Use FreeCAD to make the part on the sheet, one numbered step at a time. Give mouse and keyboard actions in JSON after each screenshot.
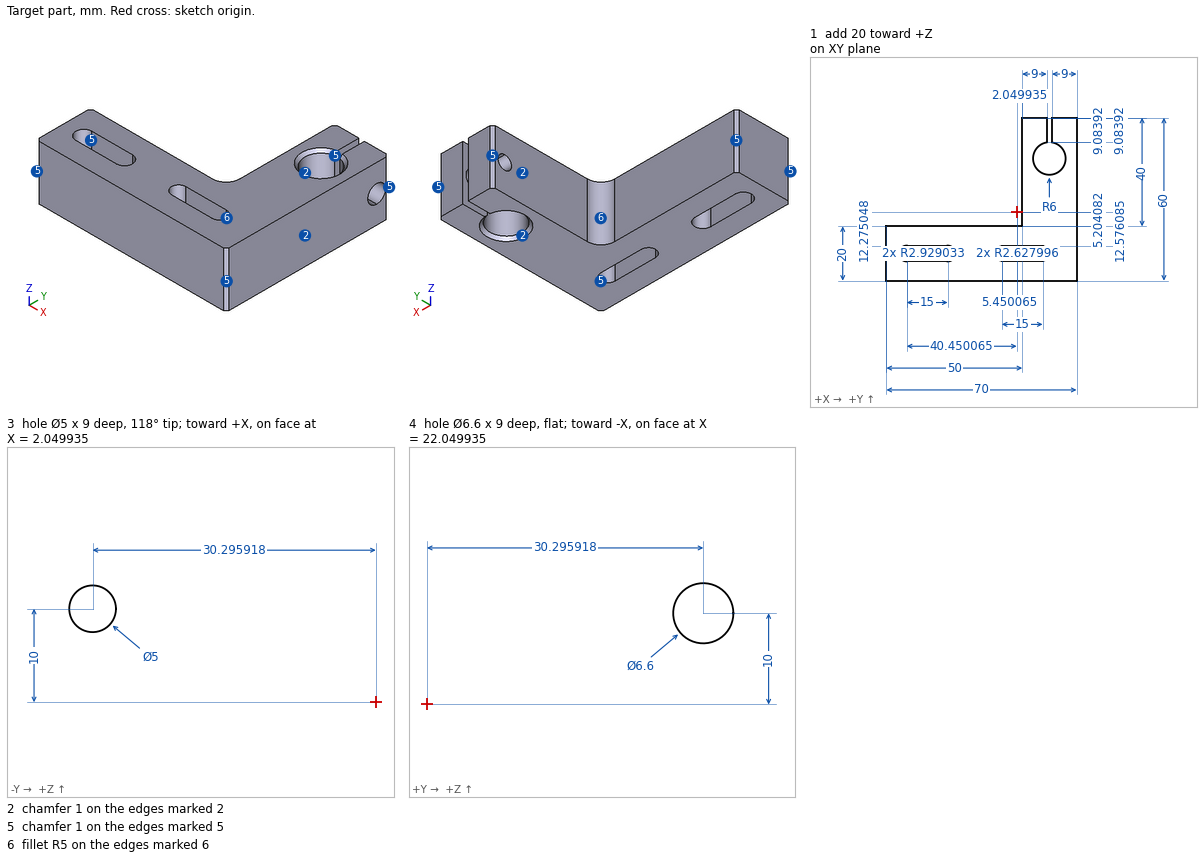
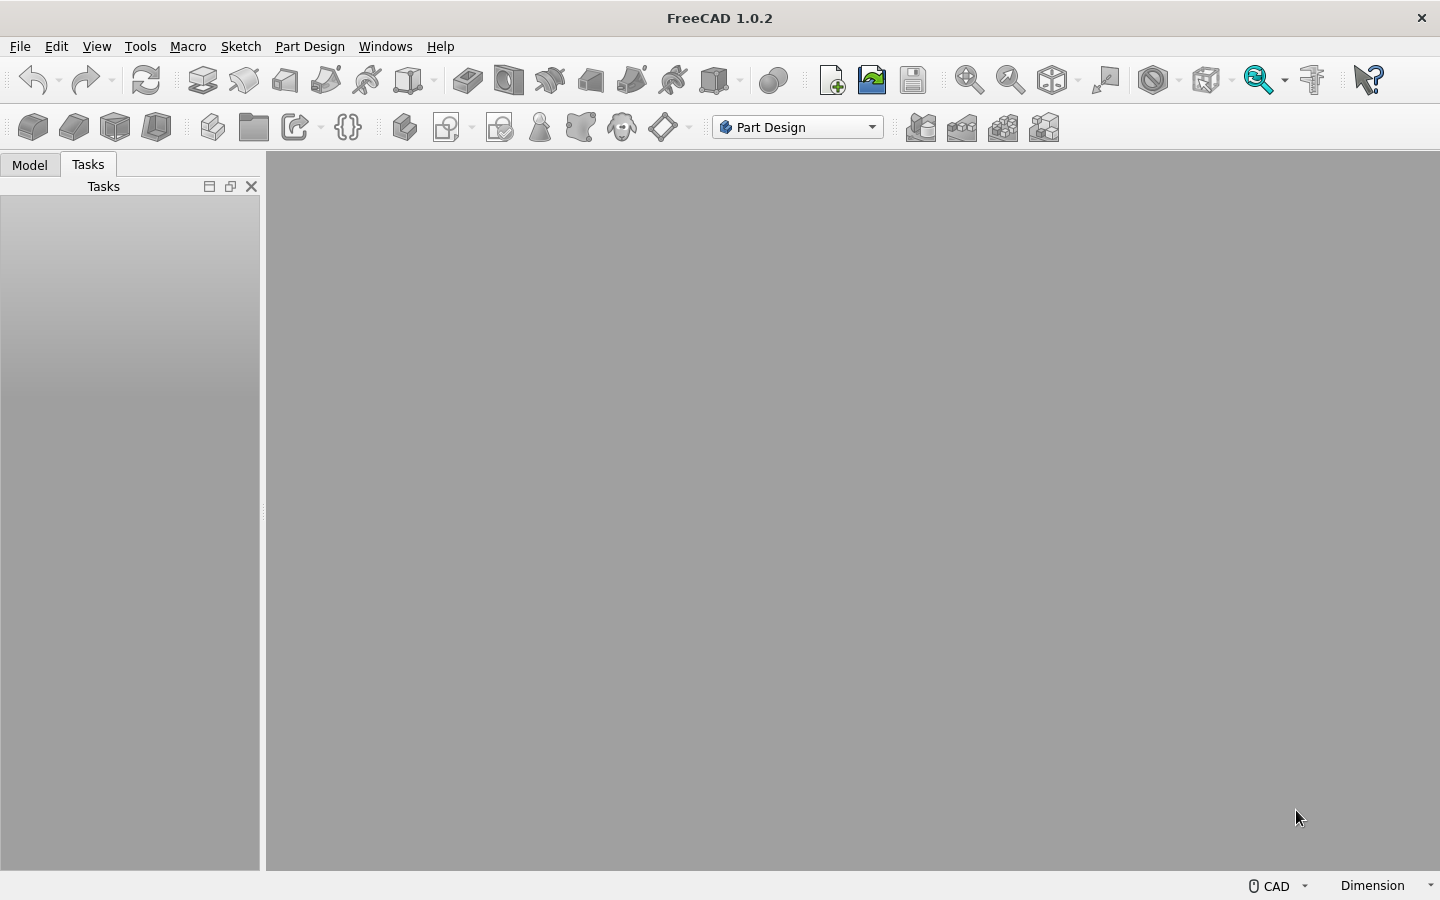
{"action": "left_click", "coordinate": [831, 80]}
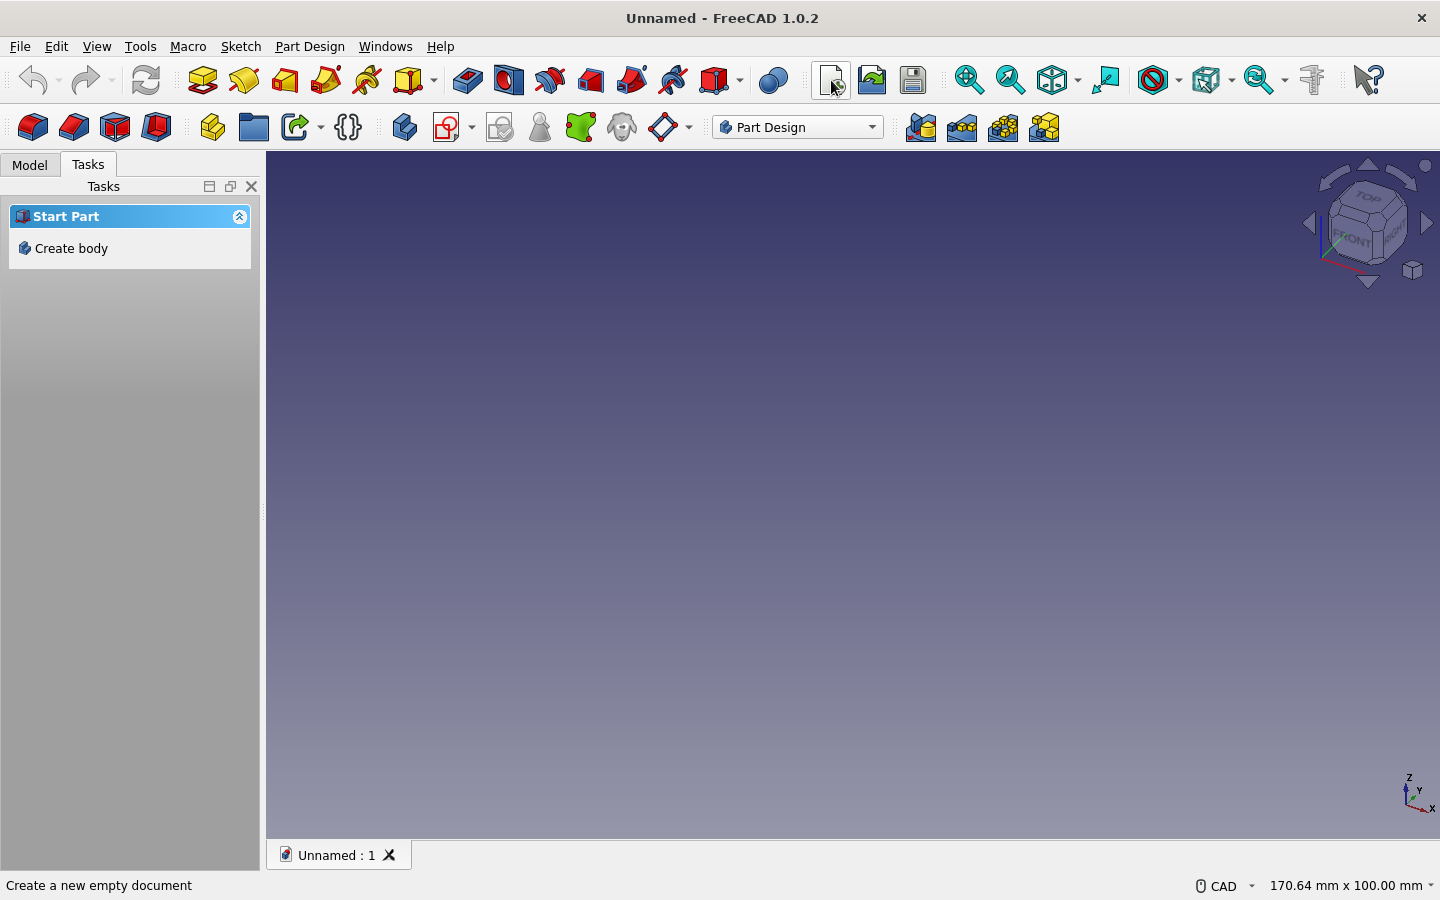
{"action": "left_click", "coordinate": [446, 128]}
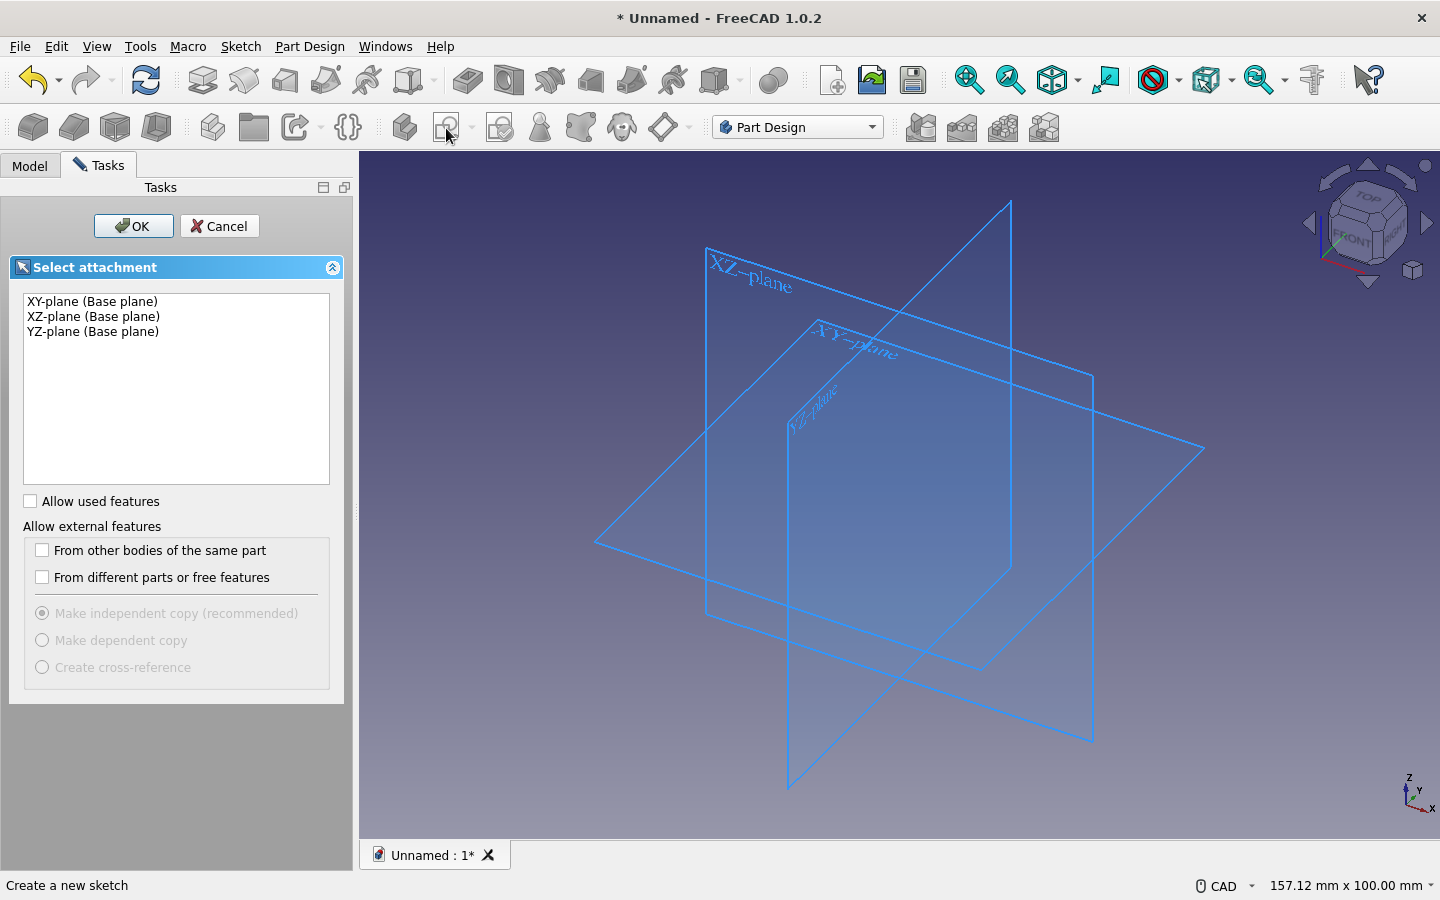
{"action": "left_click", "coordinate": [84, 302]}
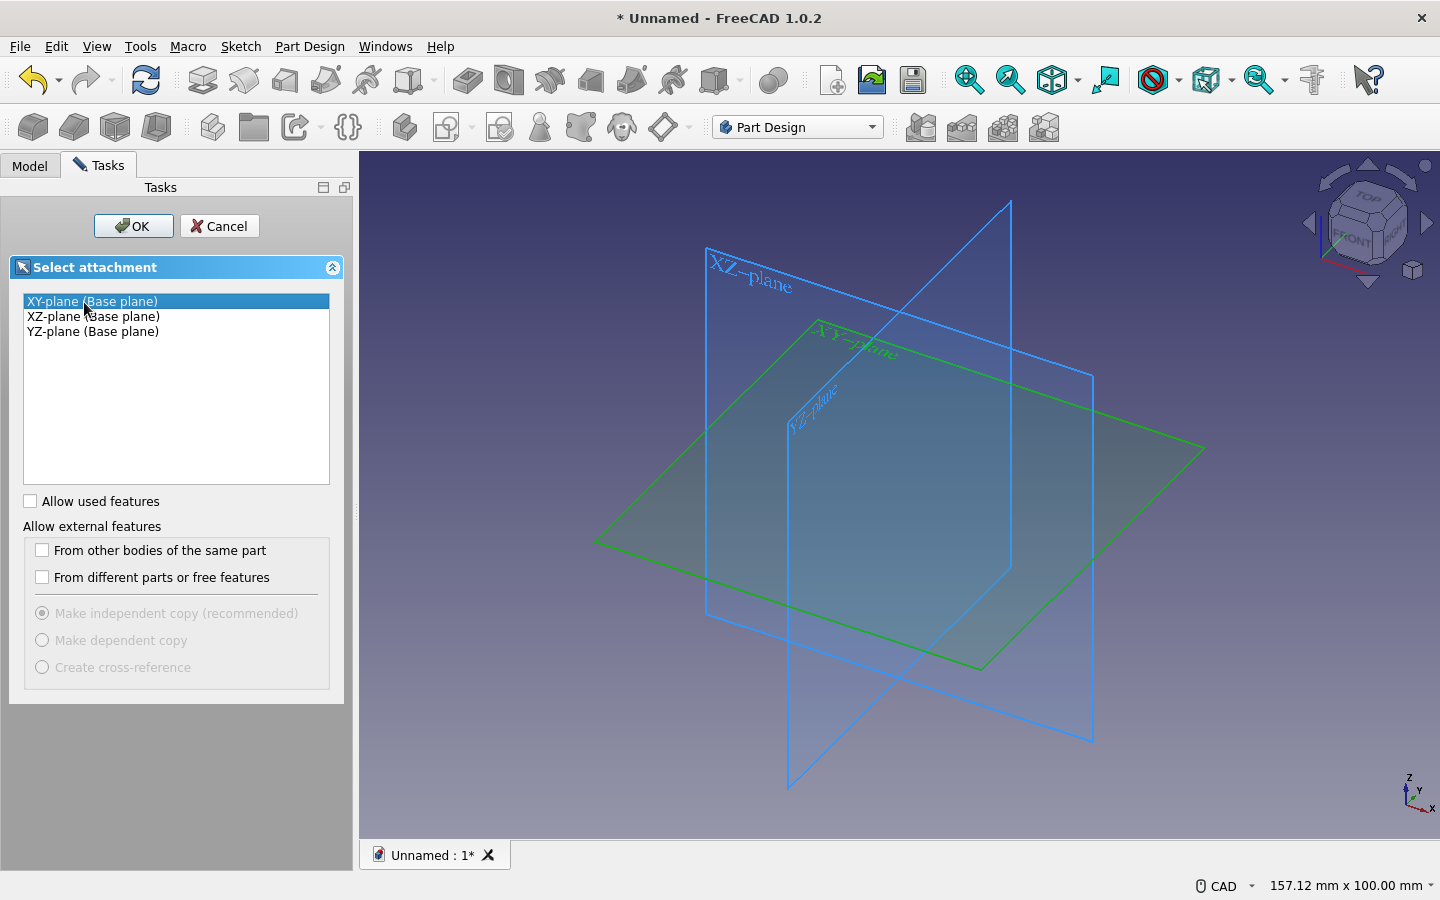
{"action": "left_click", "coordinate": [134, 226]}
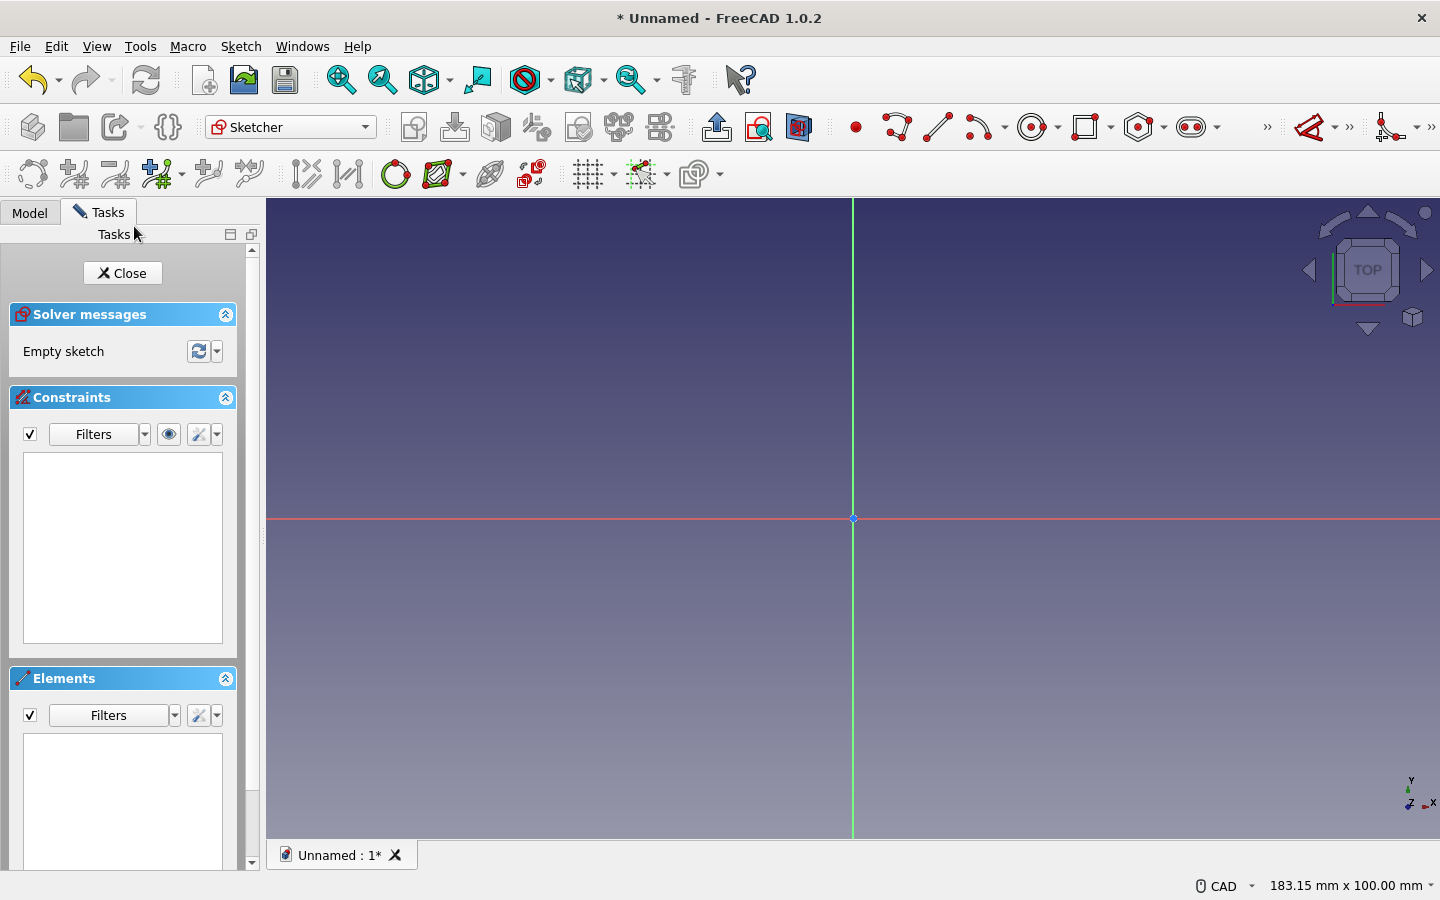
{"action": "left_click", "coordinate": [897, 128]}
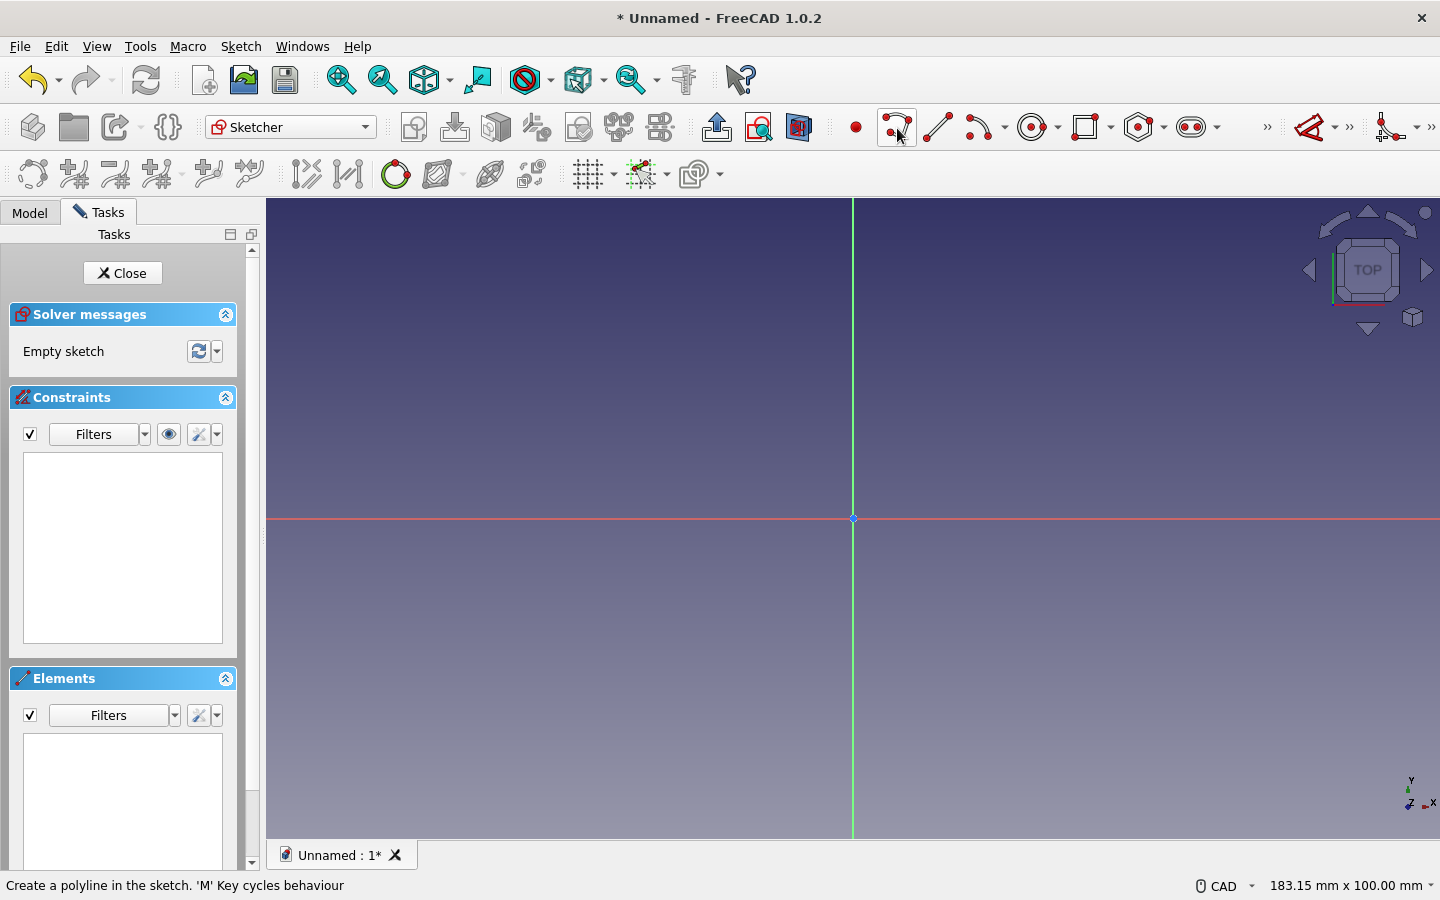
{"action": "left_click", "coordinate": [924, 354]}
{"action": "left_click", "coordinate": [924, 295]}
{"action": "left_click", "coordinate": [866, 295]}
{"action": "left_click", "coordinate": [866, 552]}
{"action": "left_click", "coordinate": [546, 552]}
{"action": "left_click", "coordinate": [546, 680]}
{"action": "left_click", "coordinate": [994, 680]}
{"action": "left_click", "coordinate": [994, 295]}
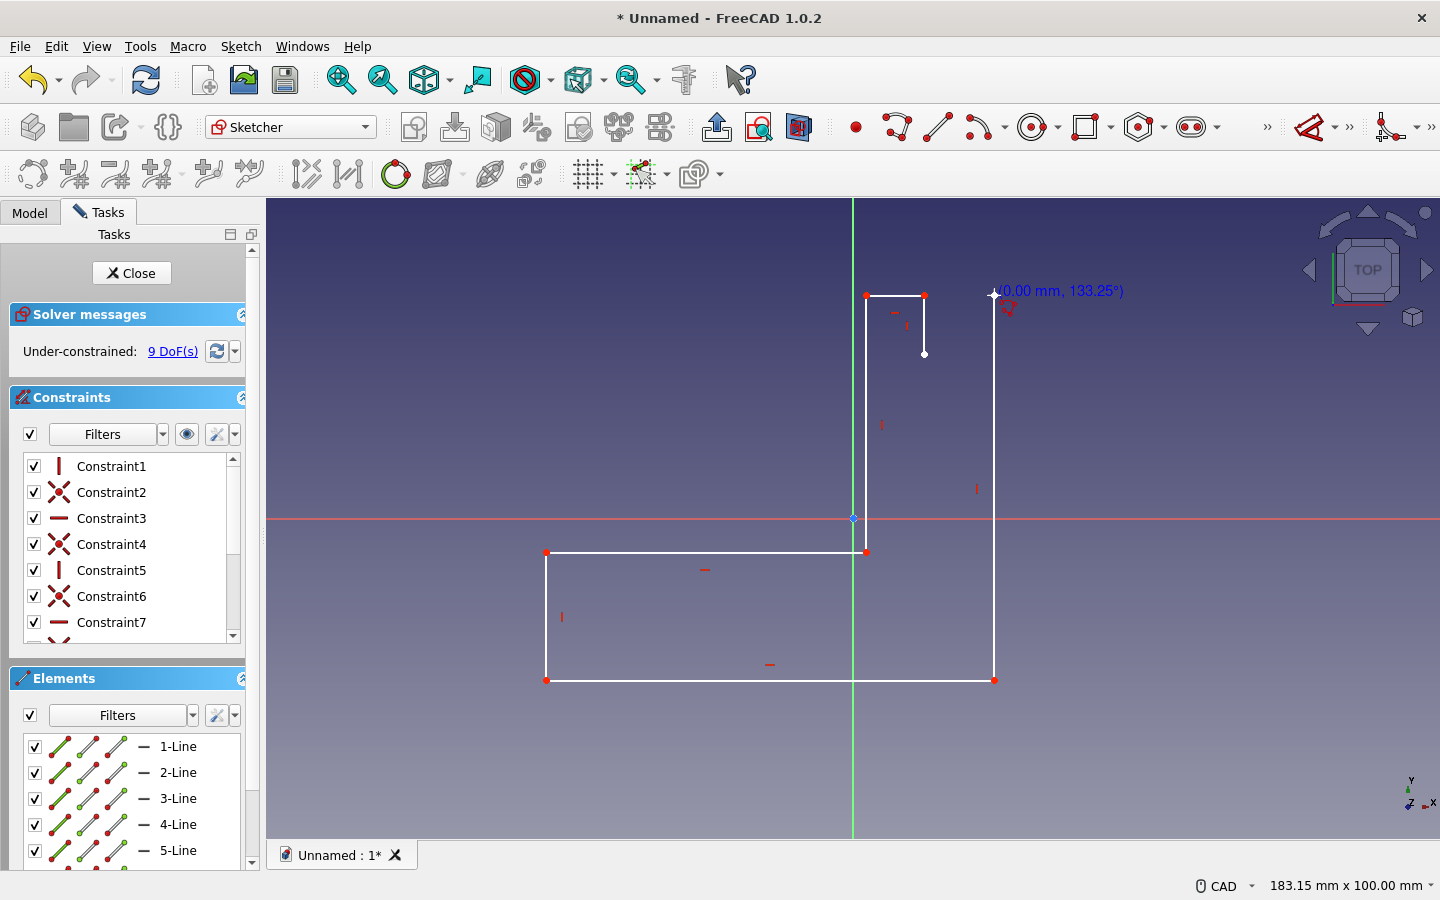
{"action": "scroll", "coordinate": [937, 295], "scroll_direction": "up", "scroll_amount": 2}